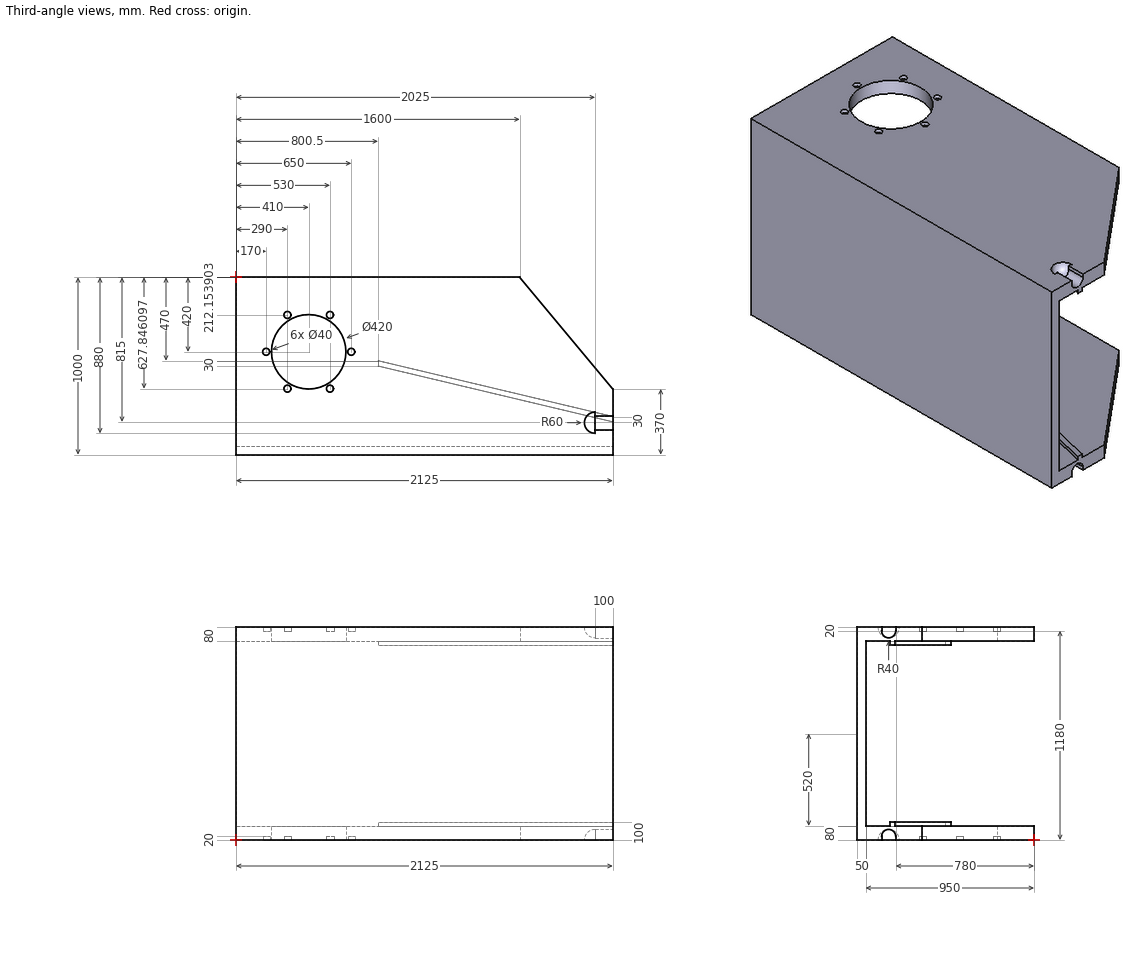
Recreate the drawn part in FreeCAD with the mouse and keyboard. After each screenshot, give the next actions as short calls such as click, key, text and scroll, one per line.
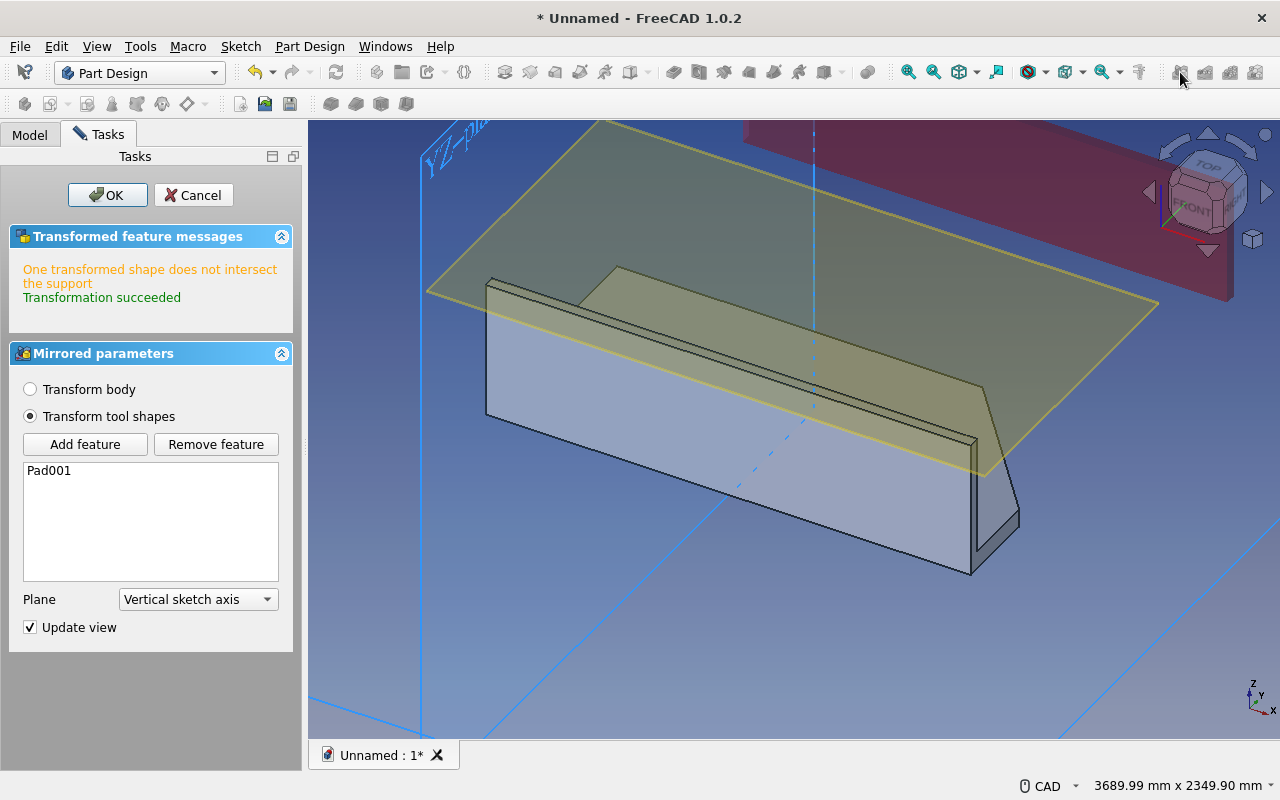
click(199, 600)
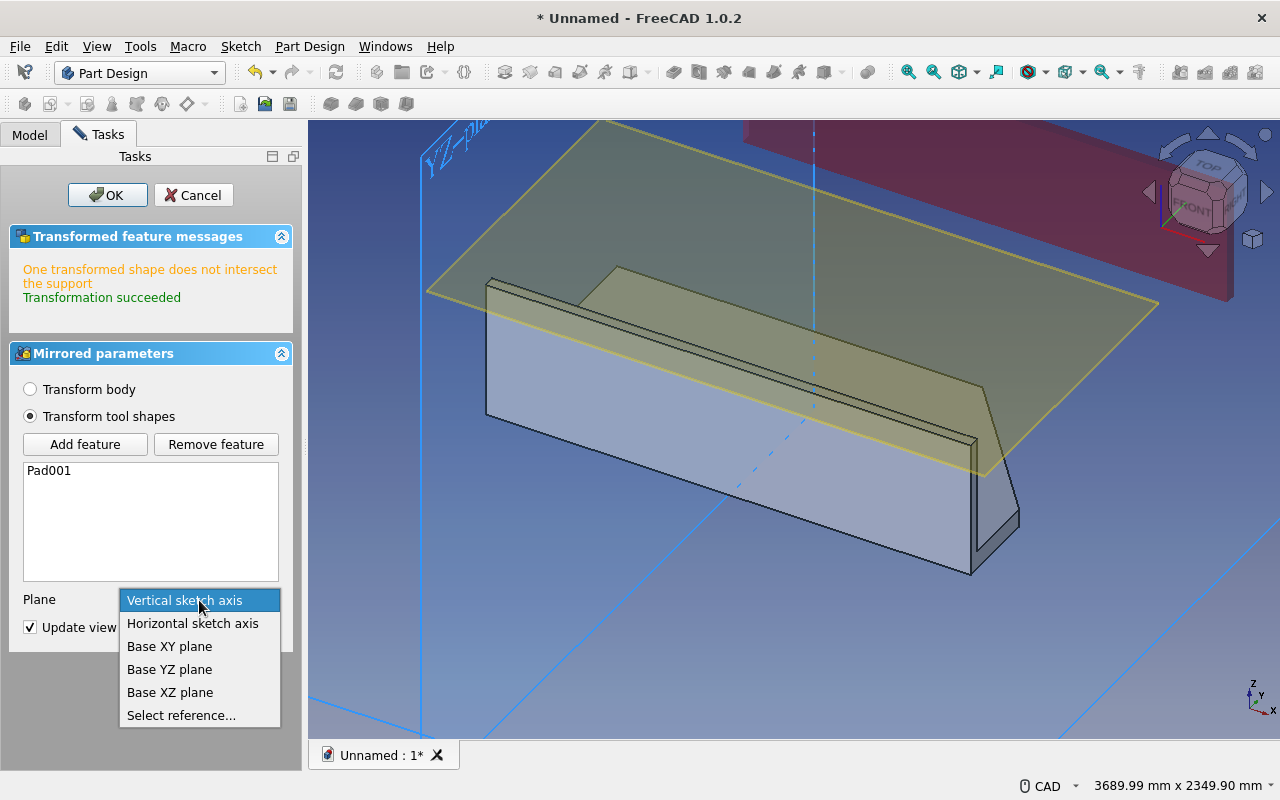
click(198, 716)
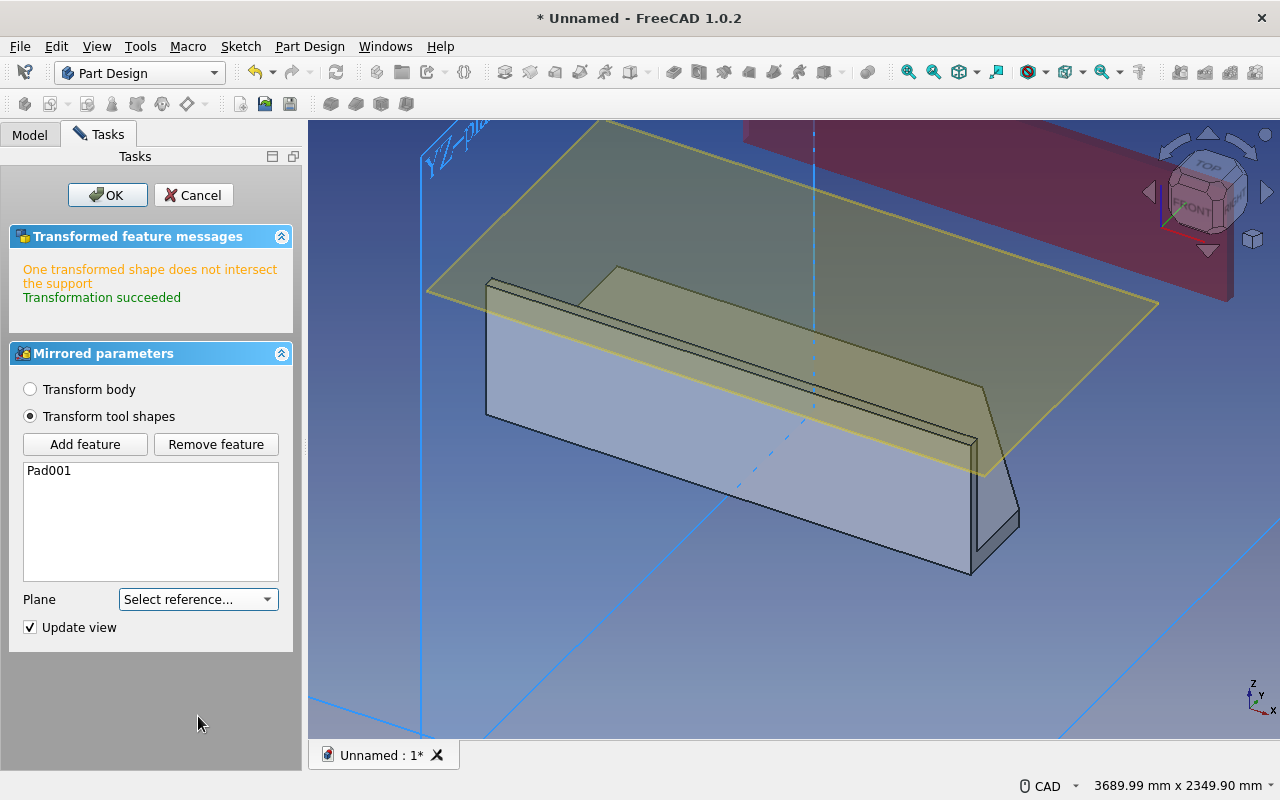
click(30, 134)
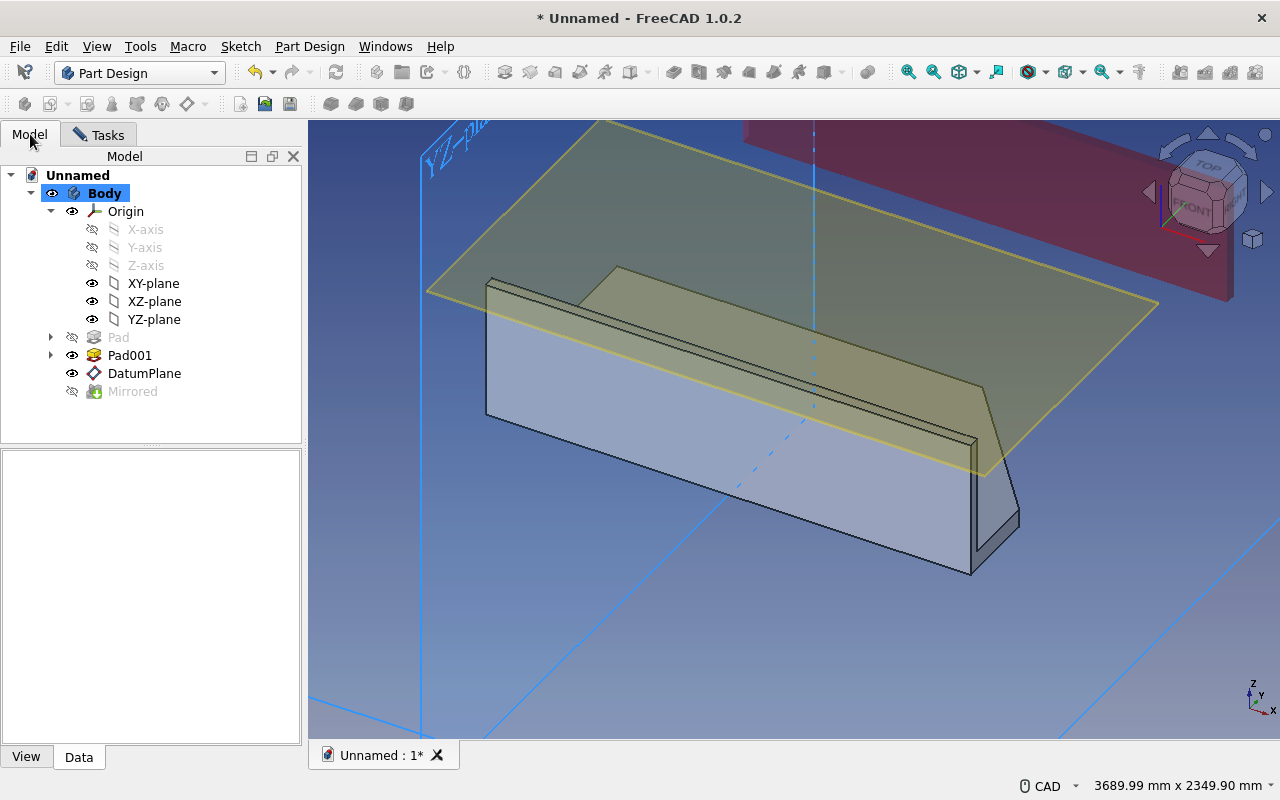
click(117, 373)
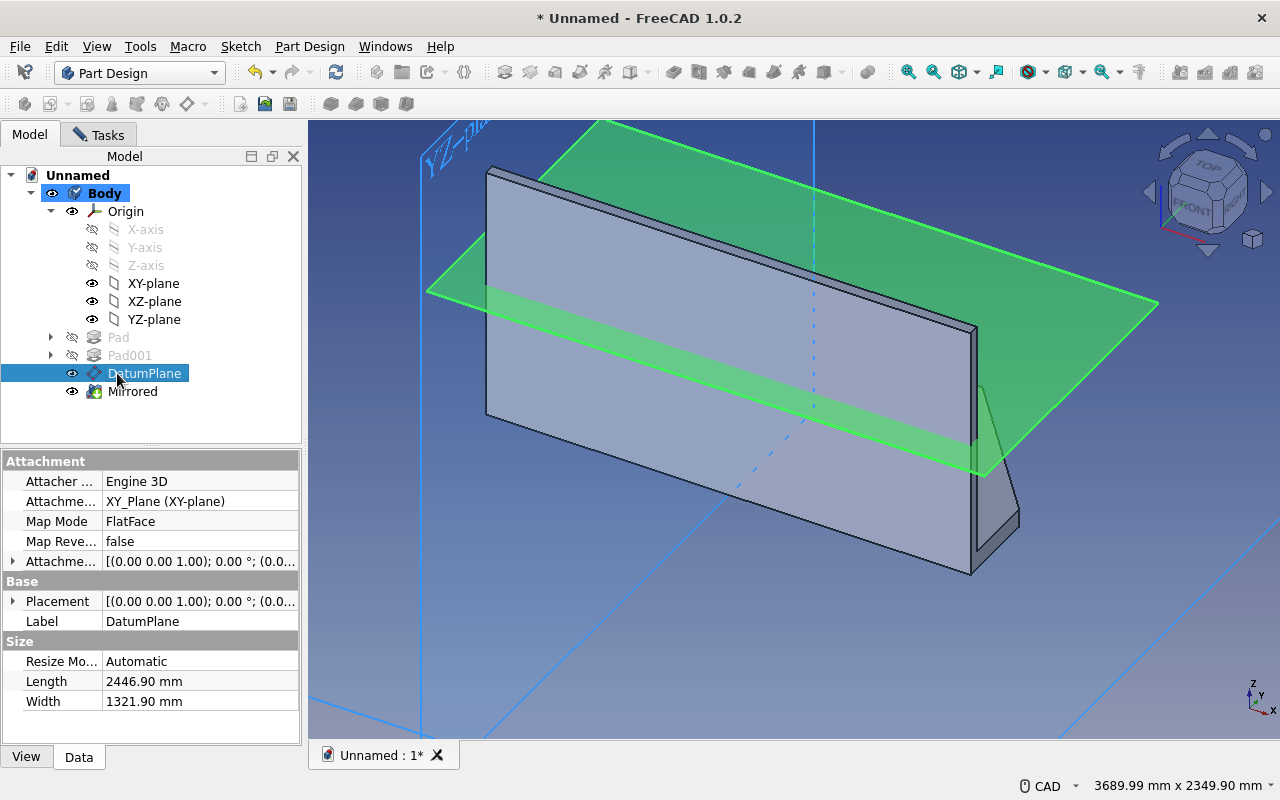
click(98, 134)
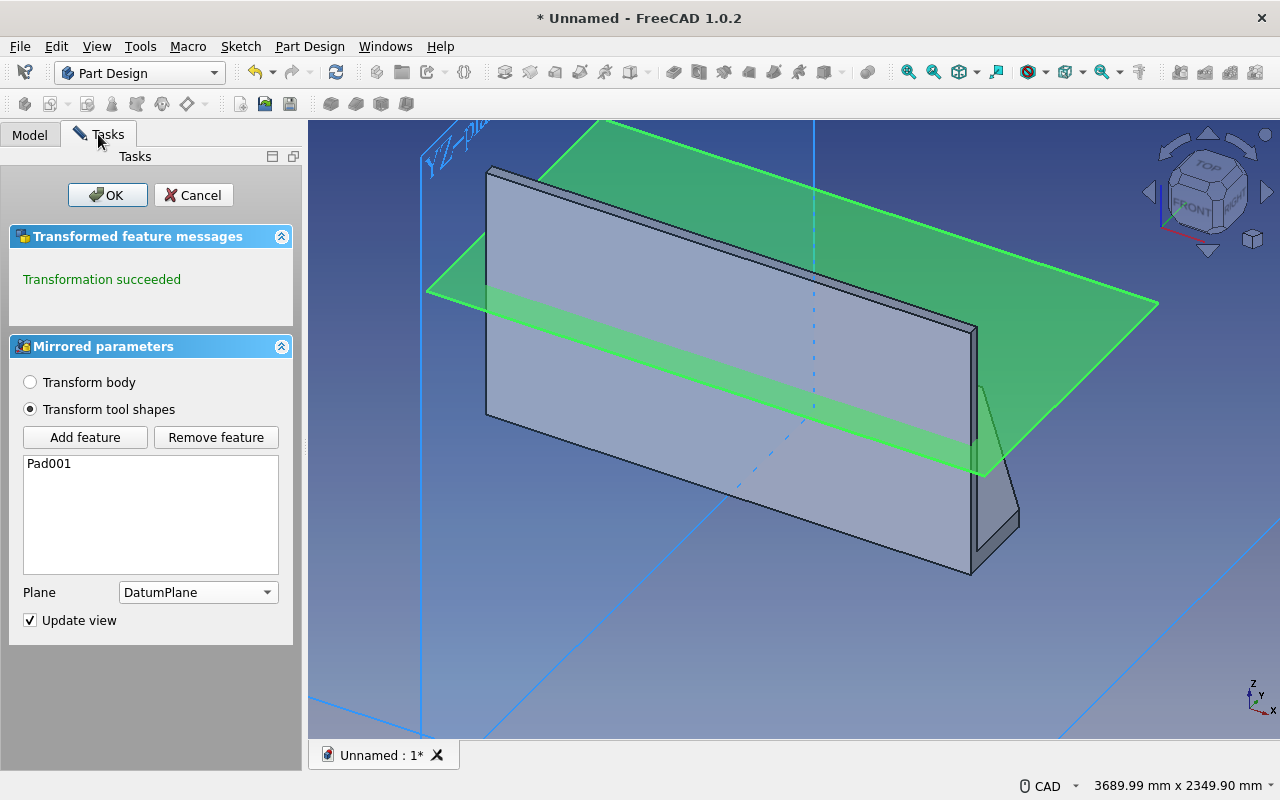
click(108, 195)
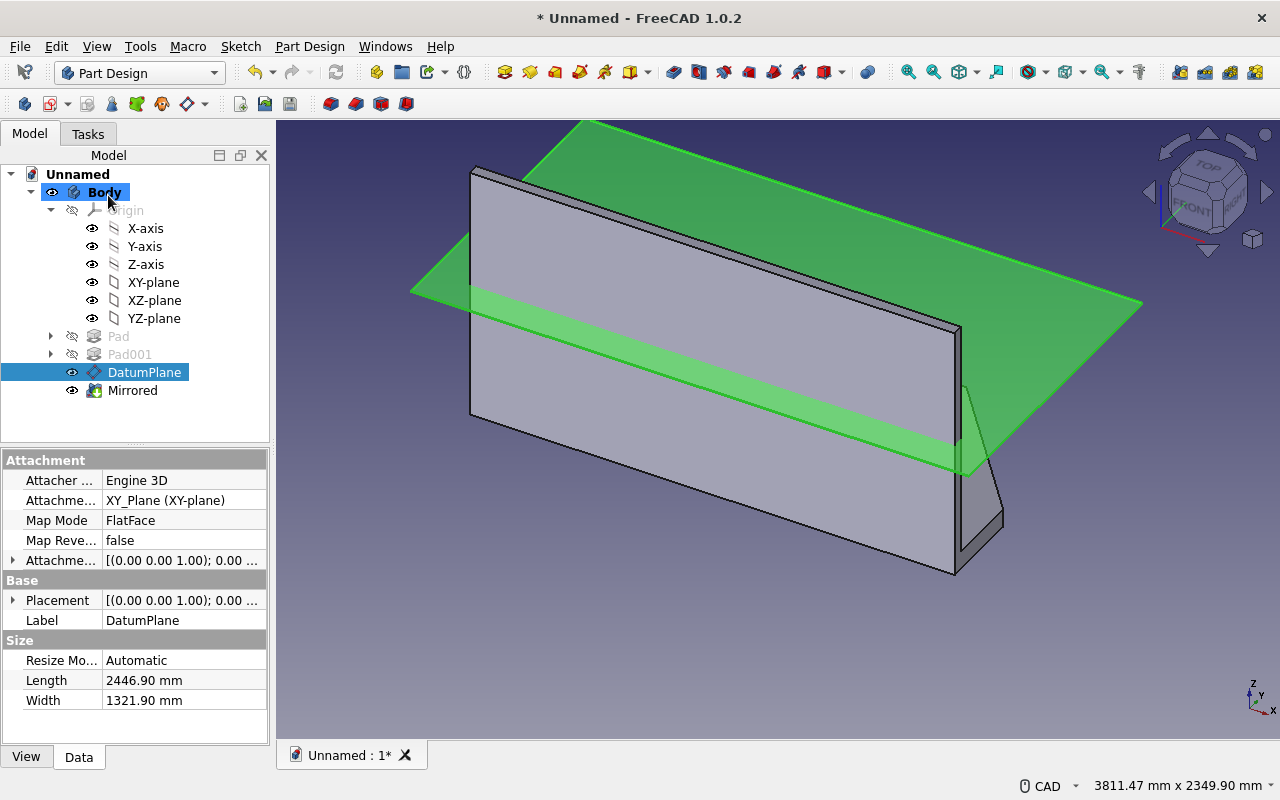
click(117, 372)
key(space)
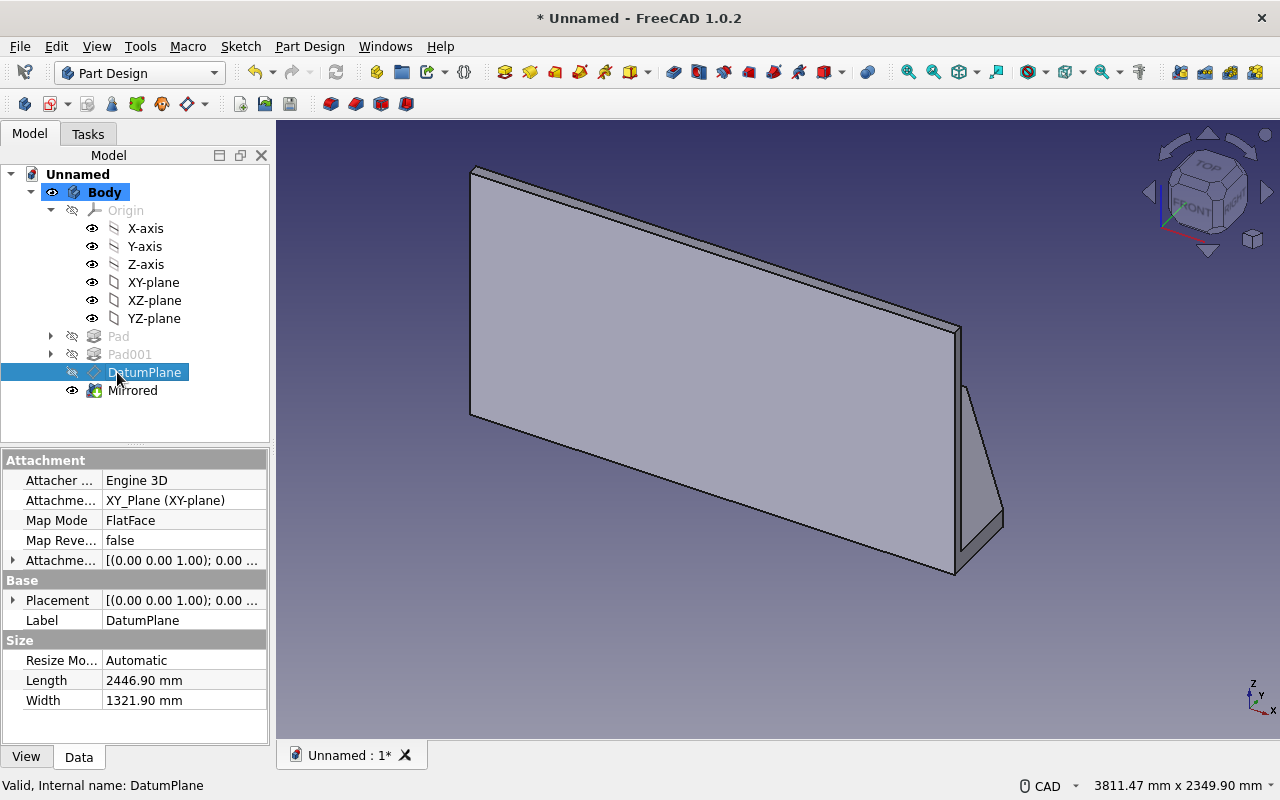
key(v)
key(f)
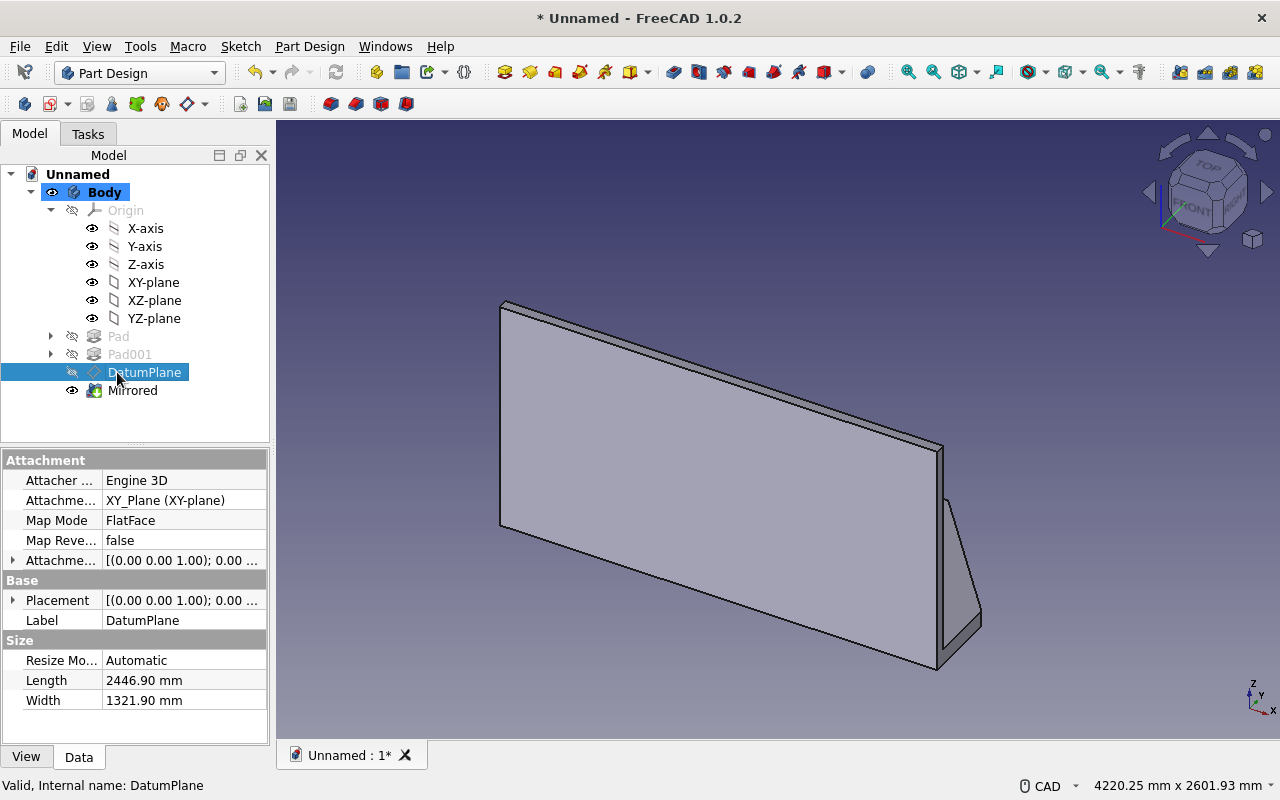
scroll(909, 438, up, 4)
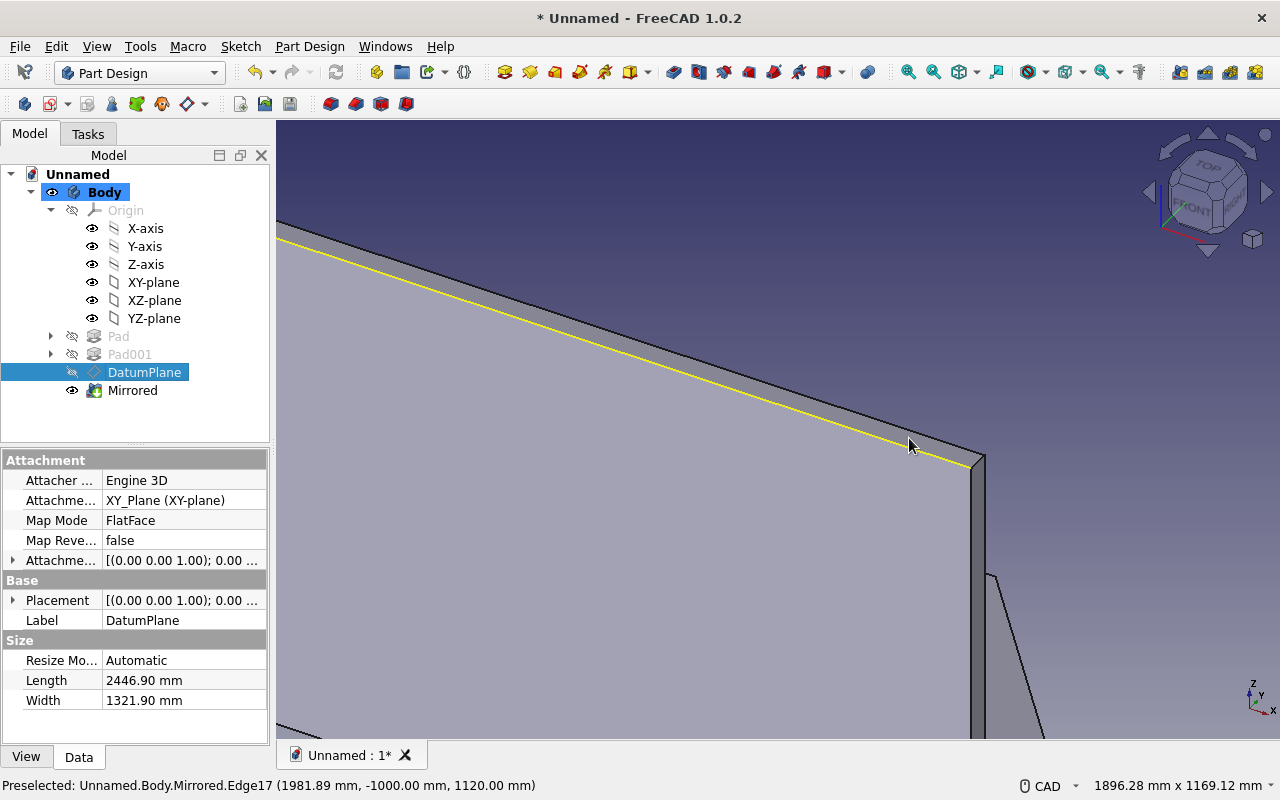
click(910, 436)